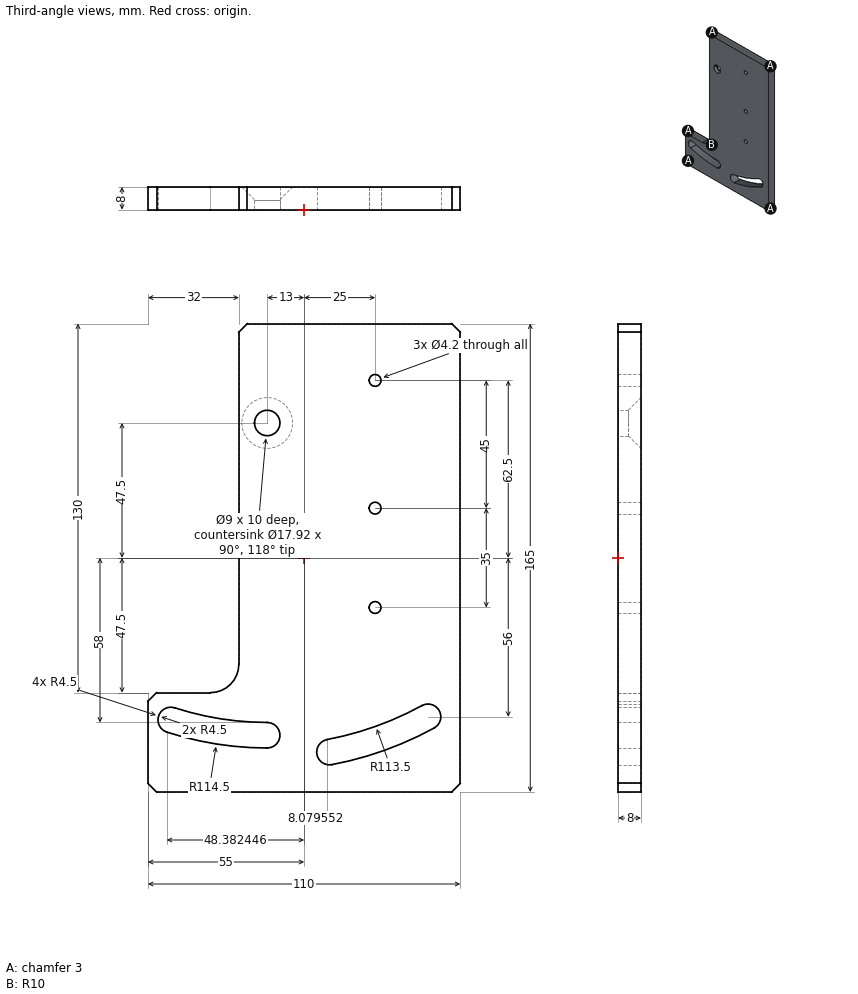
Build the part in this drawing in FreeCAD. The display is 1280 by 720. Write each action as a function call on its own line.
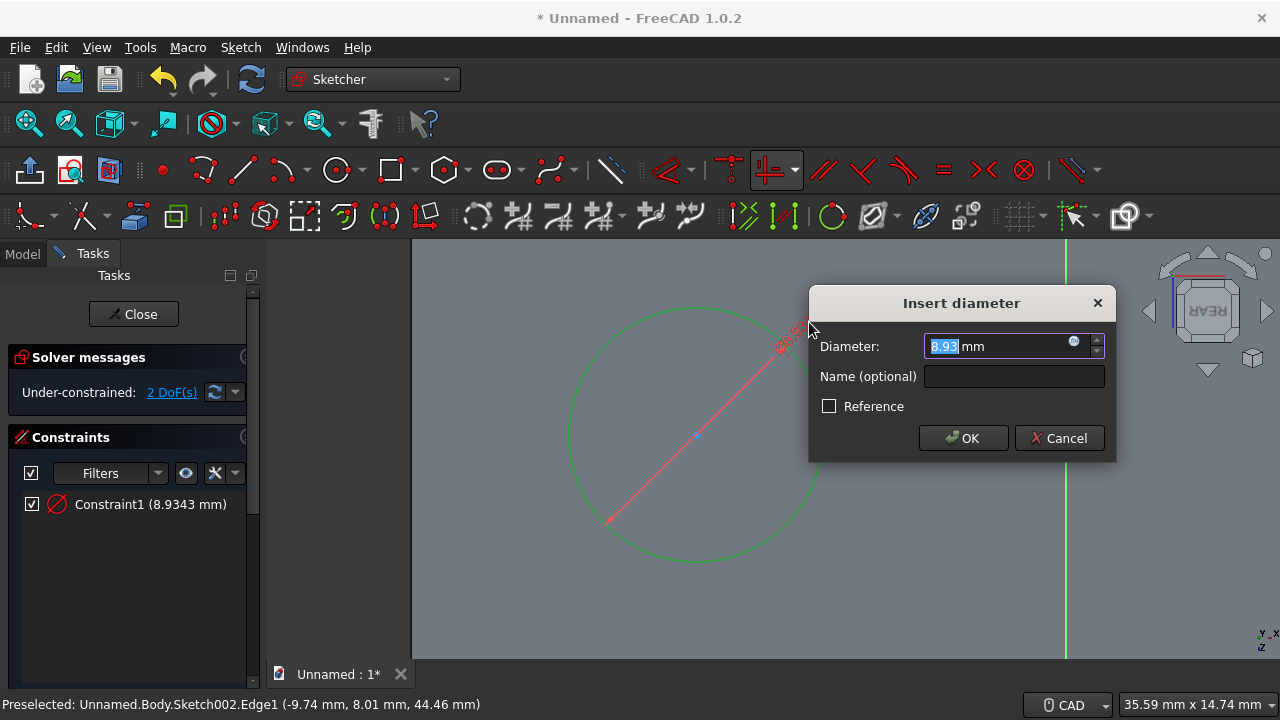
text(9)
key(Return)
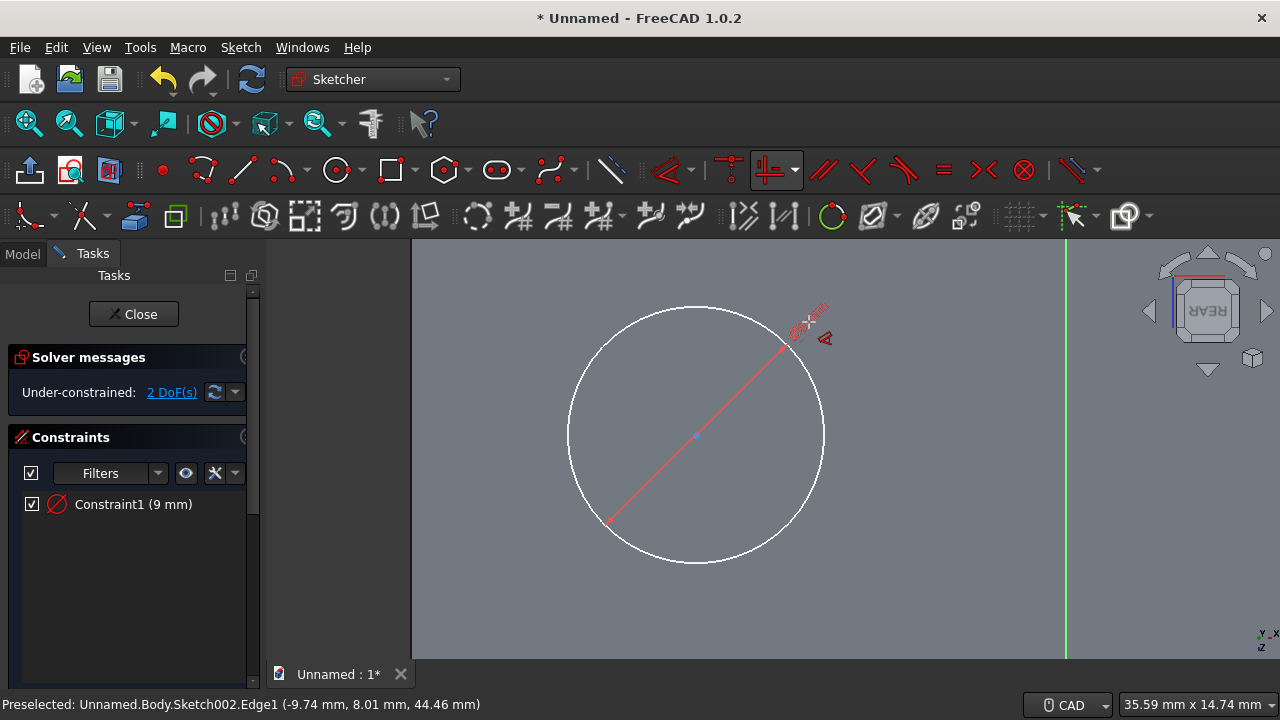
click(696, 435)
click(881, 469)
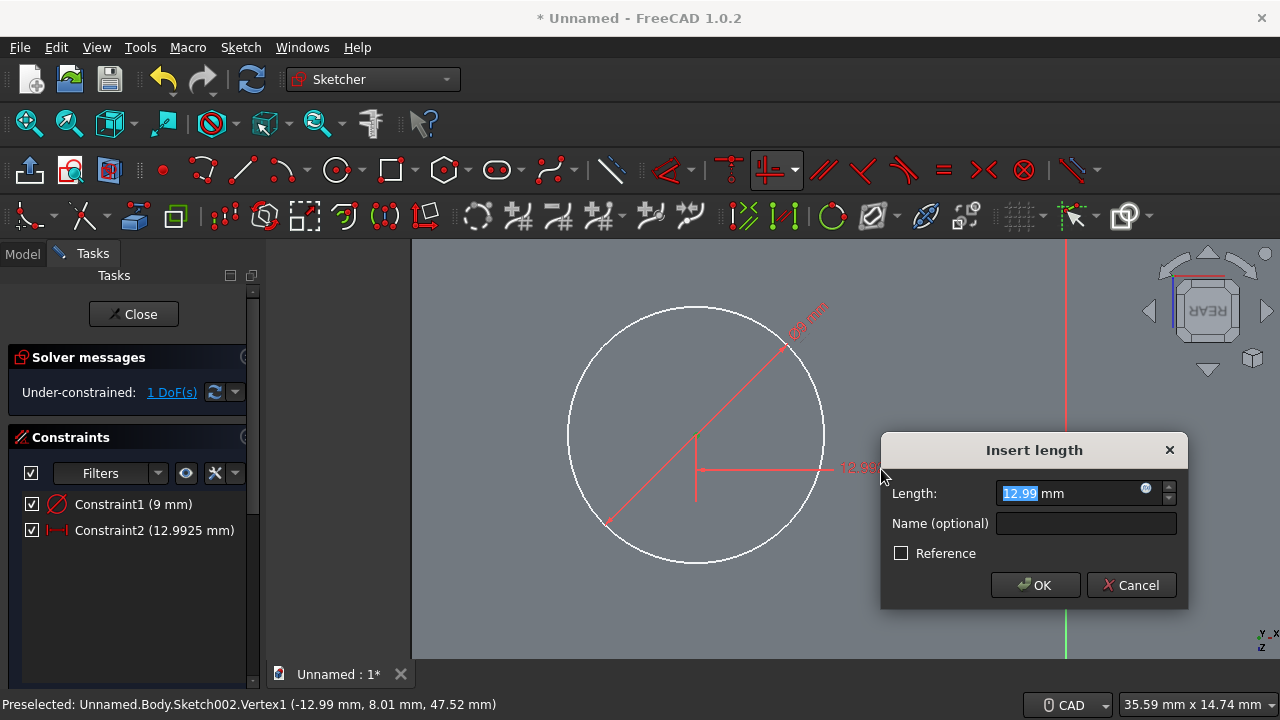
text(13)
key(Return)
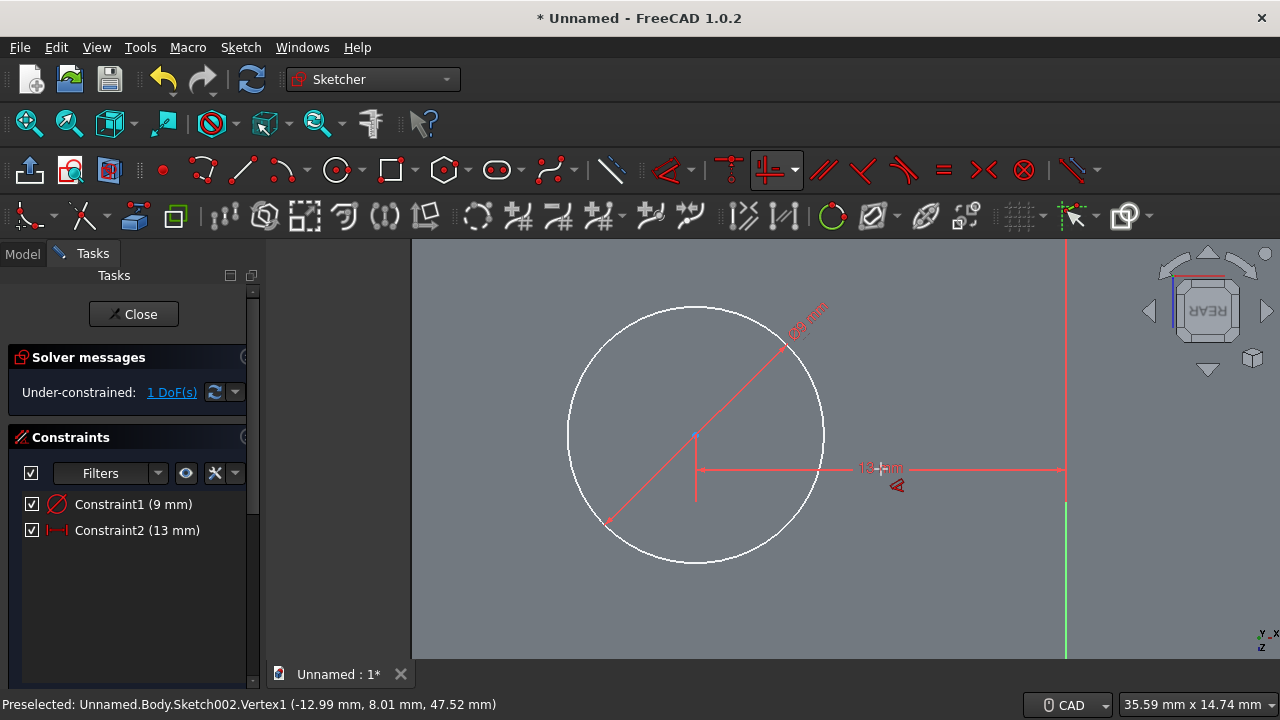
click(696, 435)
click(1100, 351)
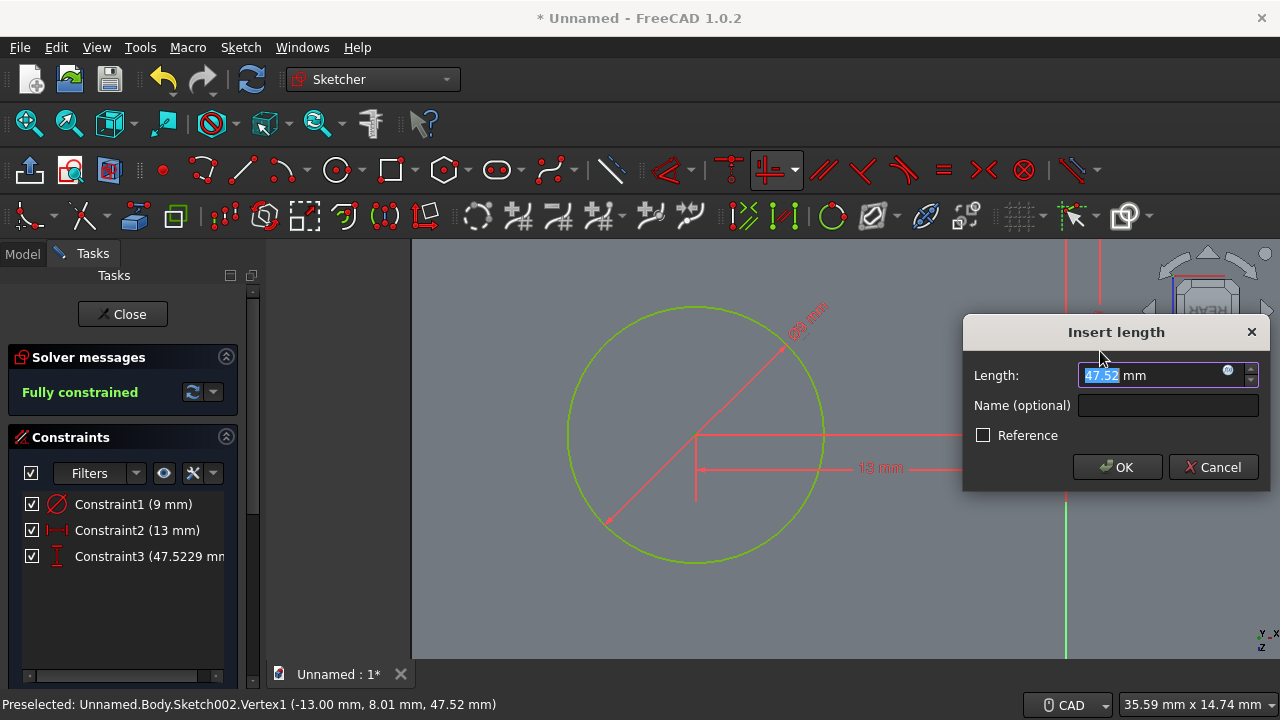
text(47.5)
key(Return)
key(Escape)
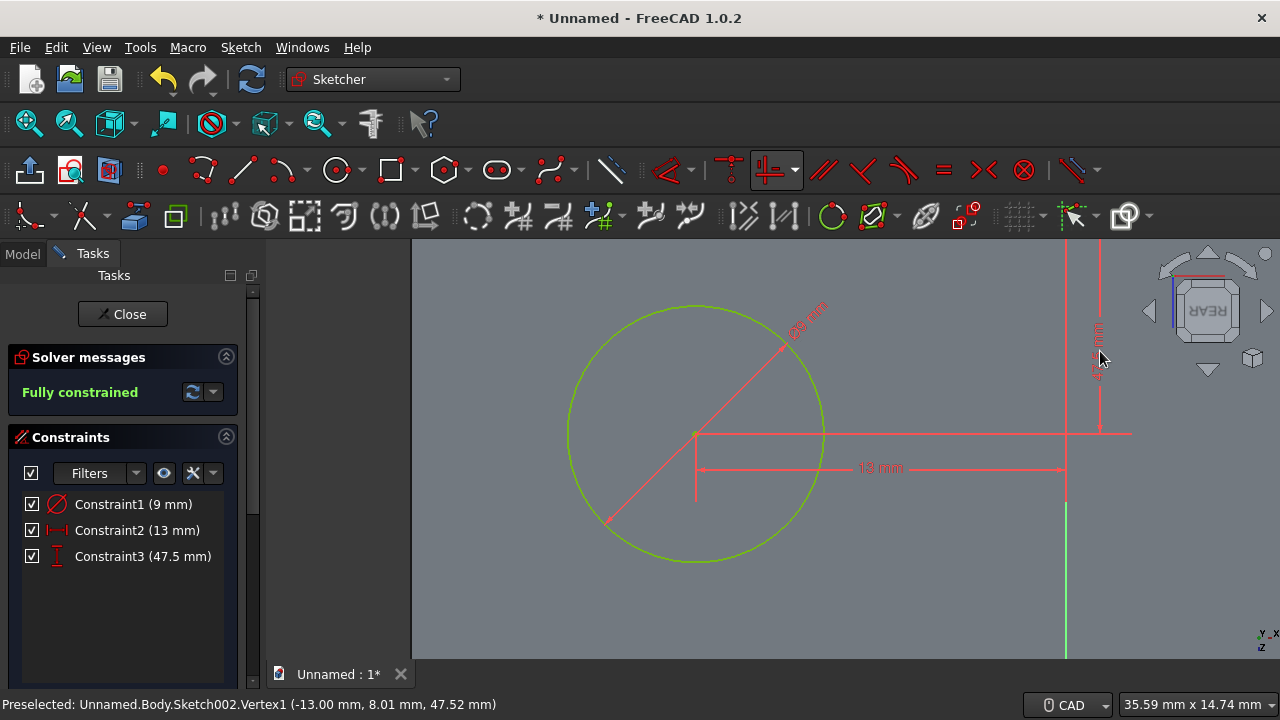
click(123, 314)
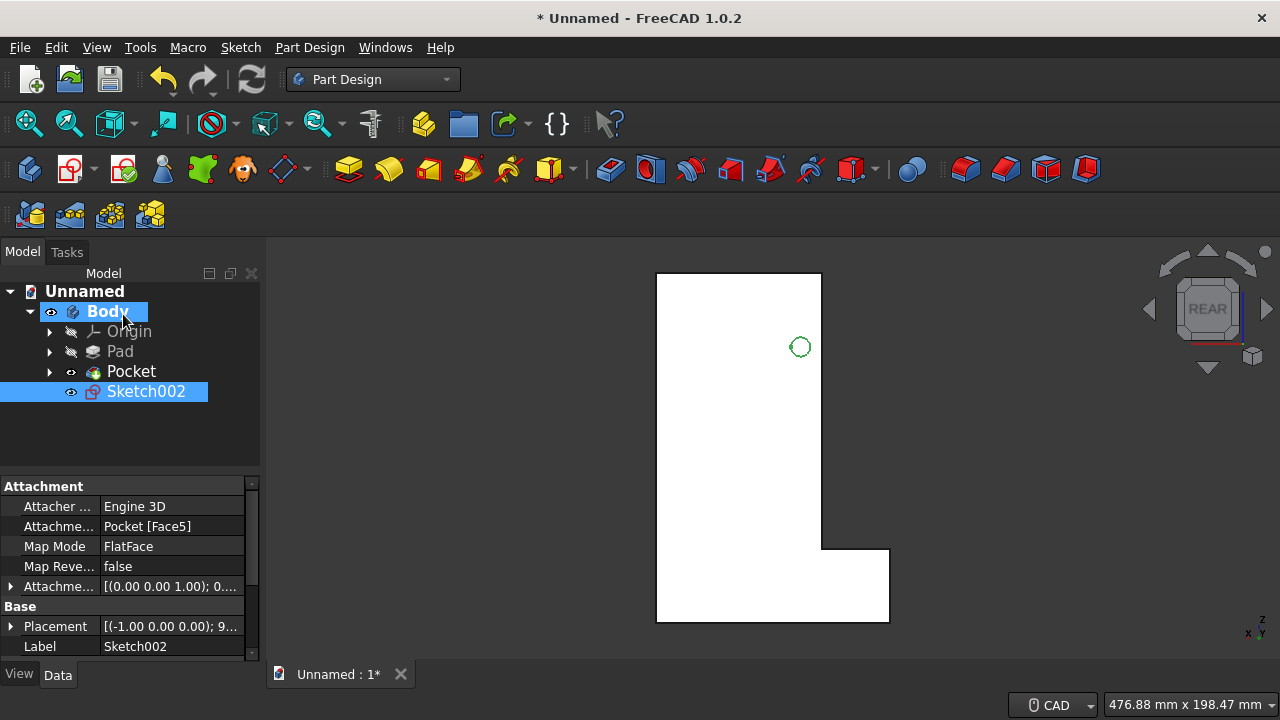
click(652, 170)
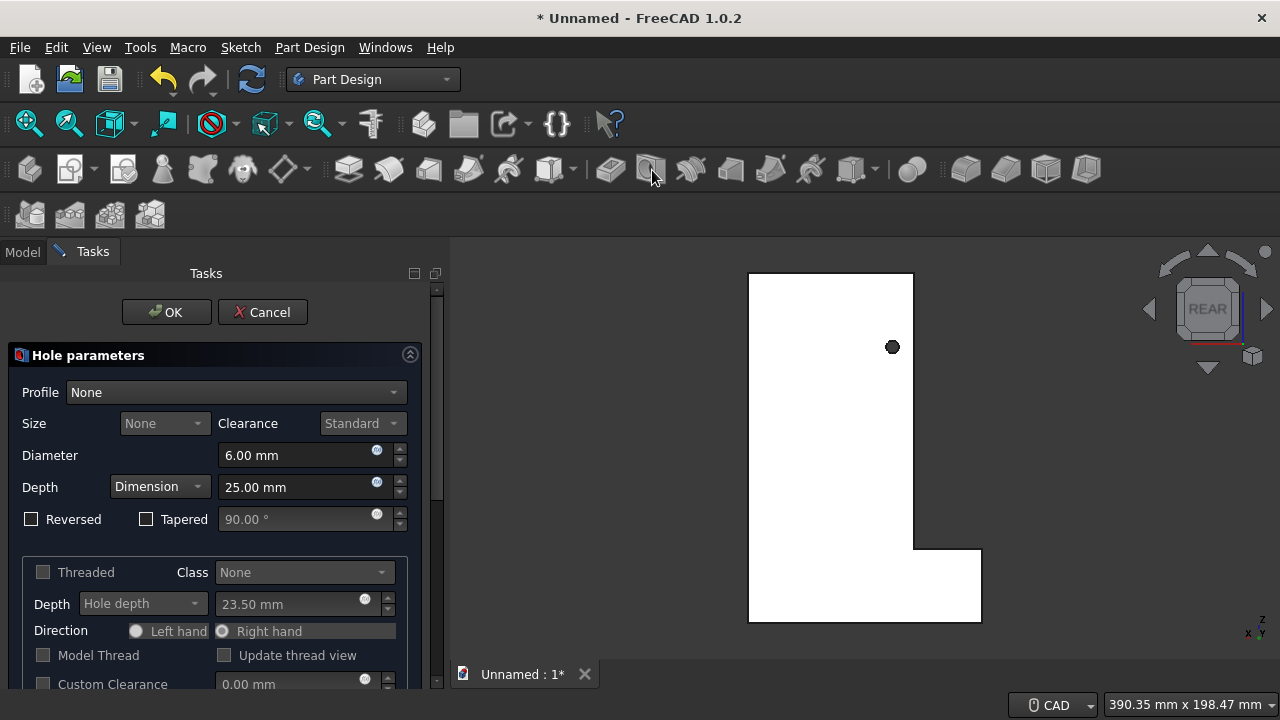
triple_click(305, 455)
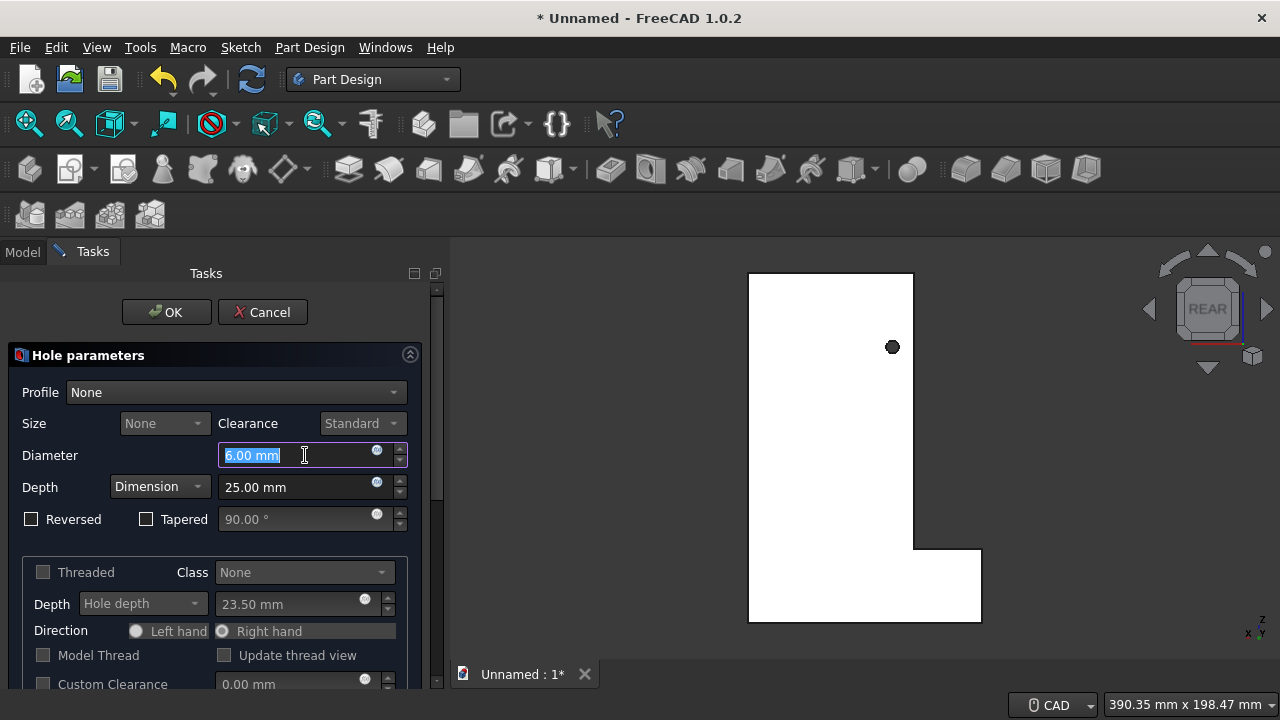
text(9)
key(Tab)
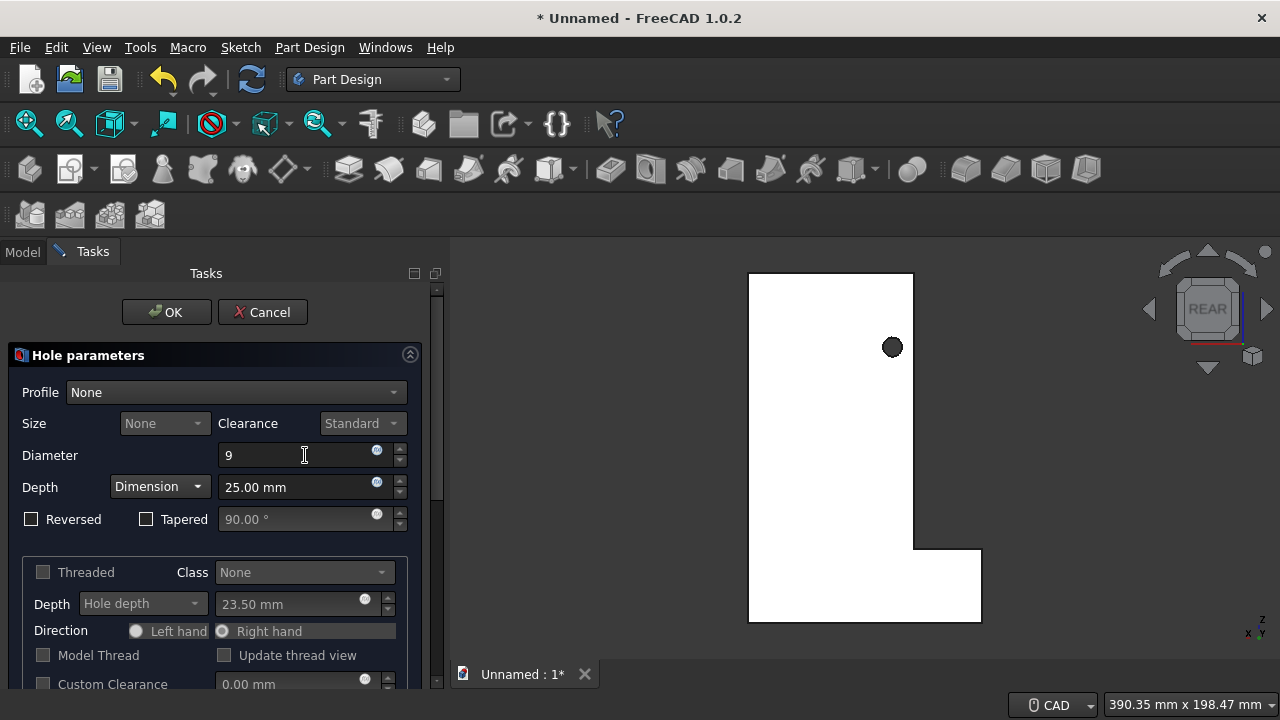
triple_click(305, 487)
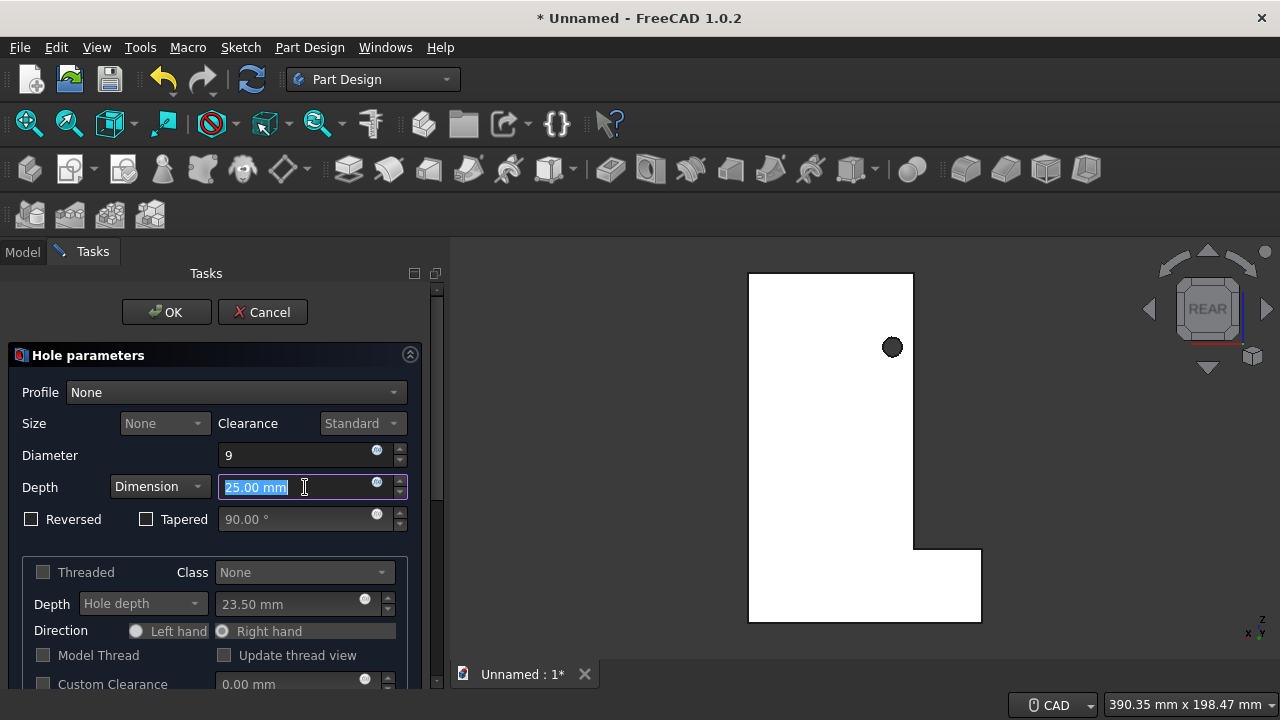
text(10)
key(Tab)